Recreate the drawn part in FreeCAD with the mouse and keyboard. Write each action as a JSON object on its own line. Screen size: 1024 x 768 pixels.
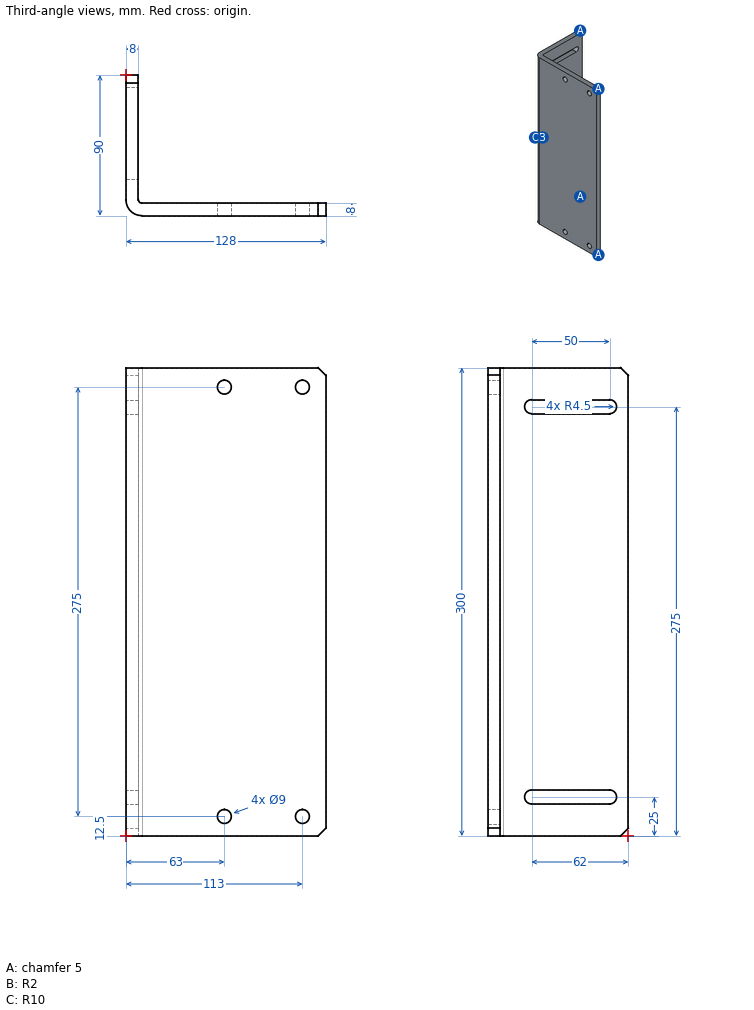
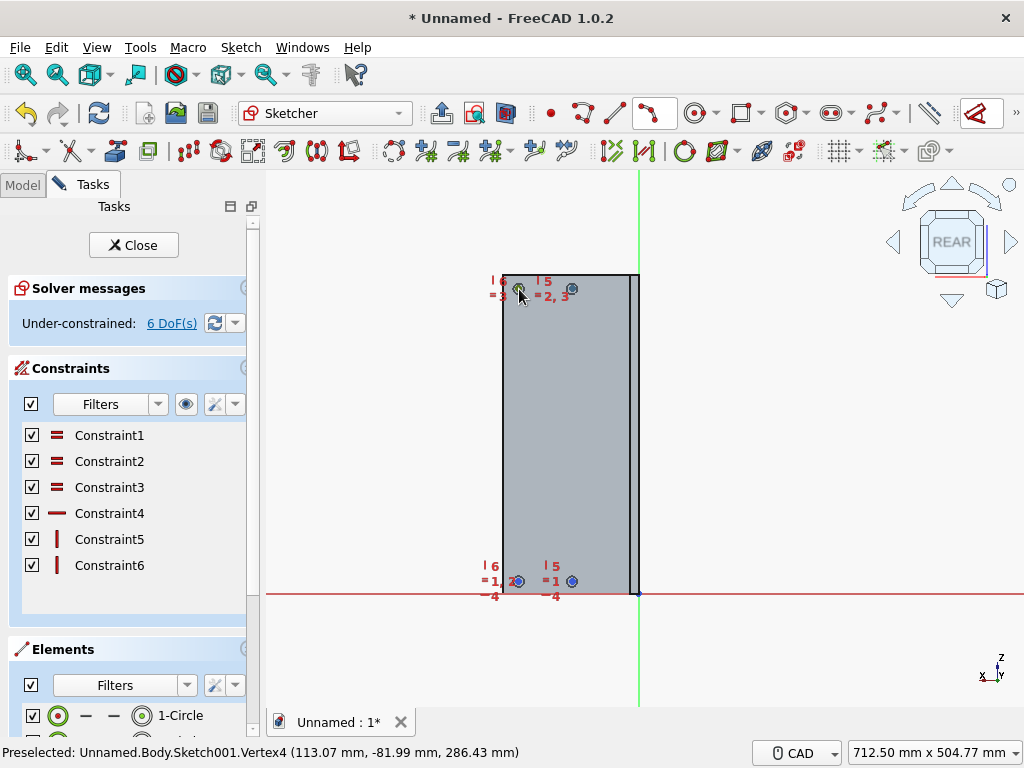
{"action": "key", "text": "h"}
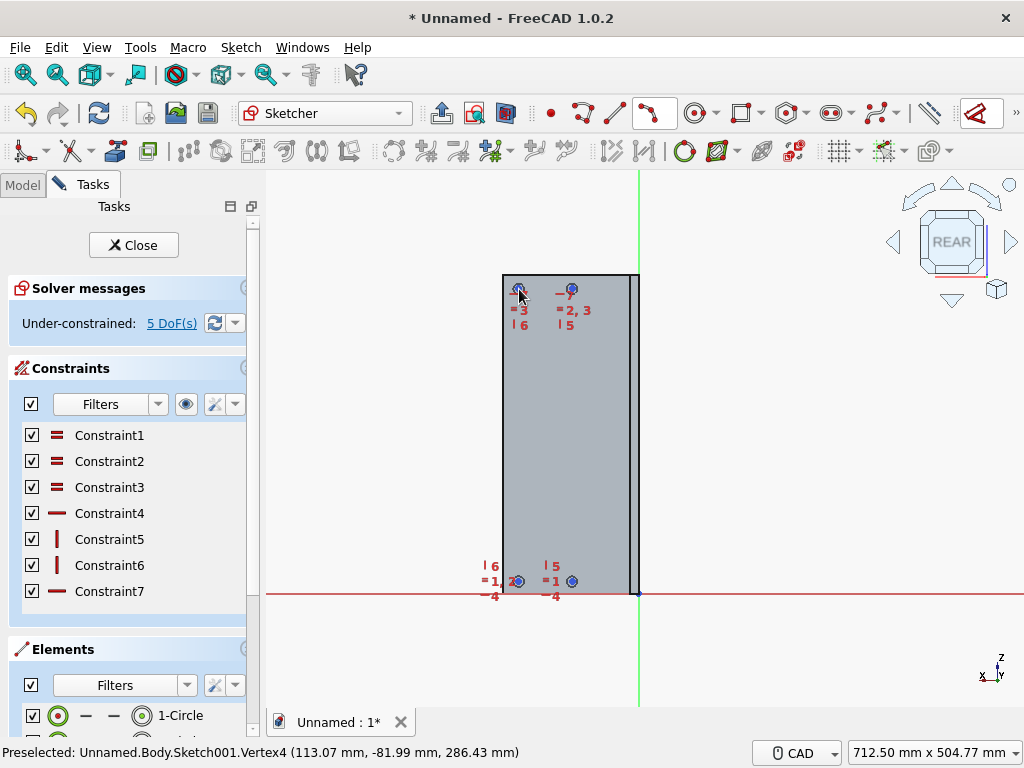
{"action": "key", "text": "d"}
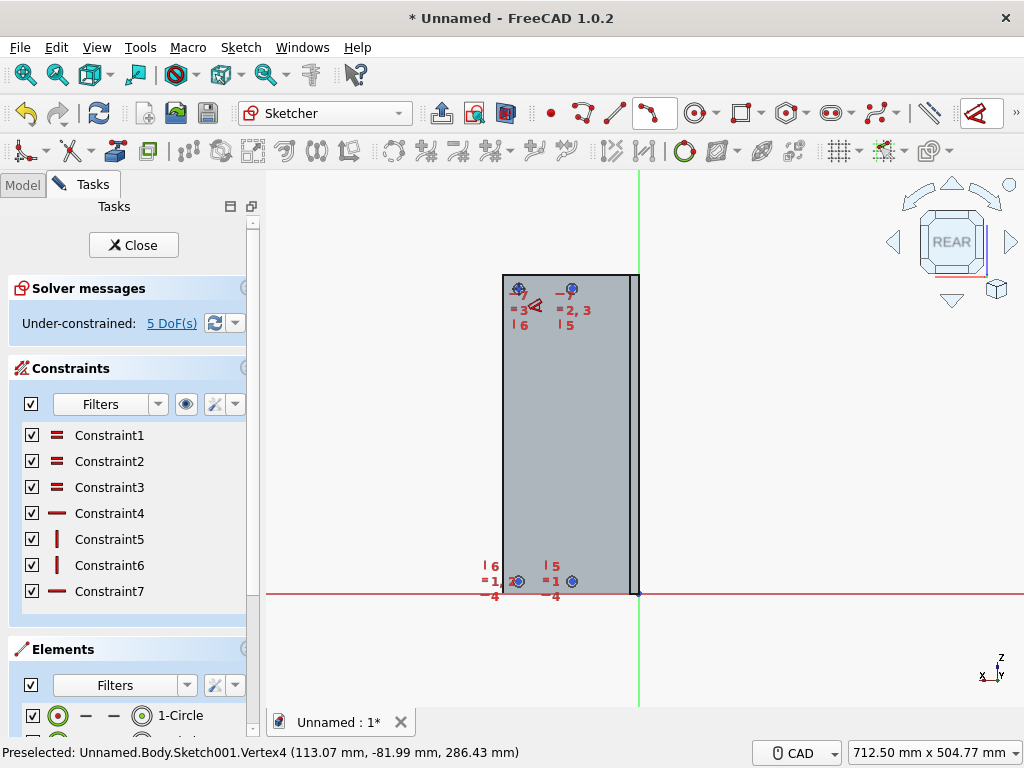
{"action": "scroll", "coordinate": [577, 582], "scroll_direction": "up", "scroll_amount": 8}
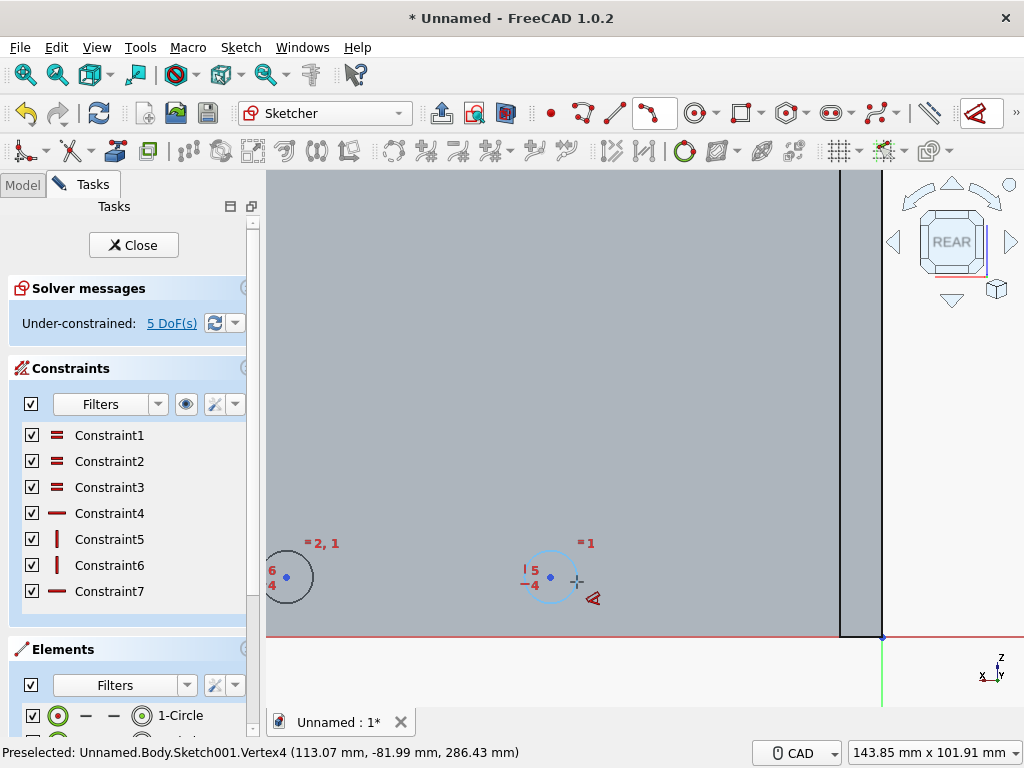
{"action": "left_click", "coordinate": [577, 578]}
{"action": "left_click", "coordinate": [609, 579]}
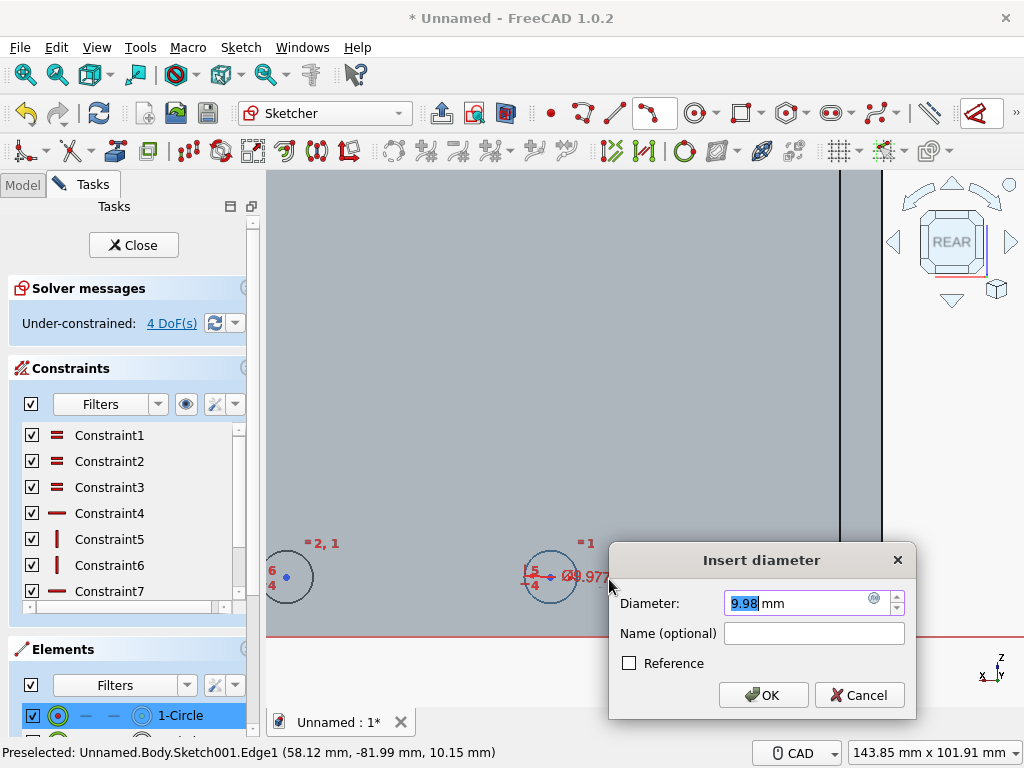
{"action": "type", "text": "9"}
{"action": "key", "text": "Return"}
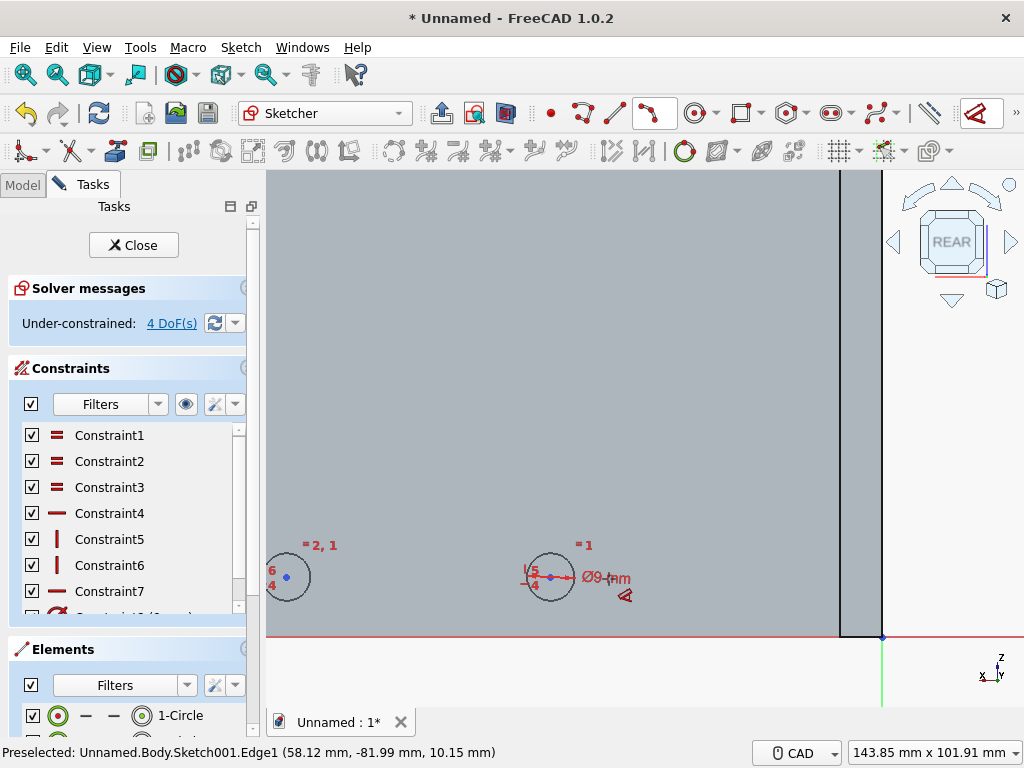
{"action": "scroll", "coordinate": [577, 583], "scroll_direction": "down", "scroll_amount": 8}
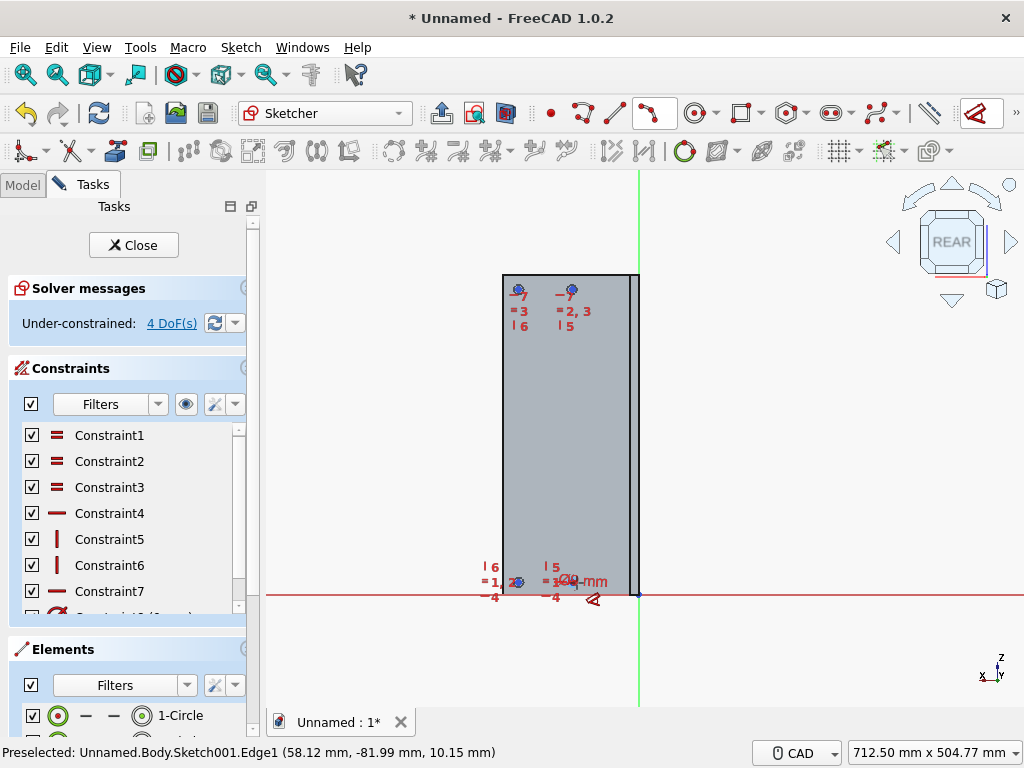
{"action": "left_click", "coordinate": [572, 582]}
{"action": "left_click", "coordinate": [606, 629]}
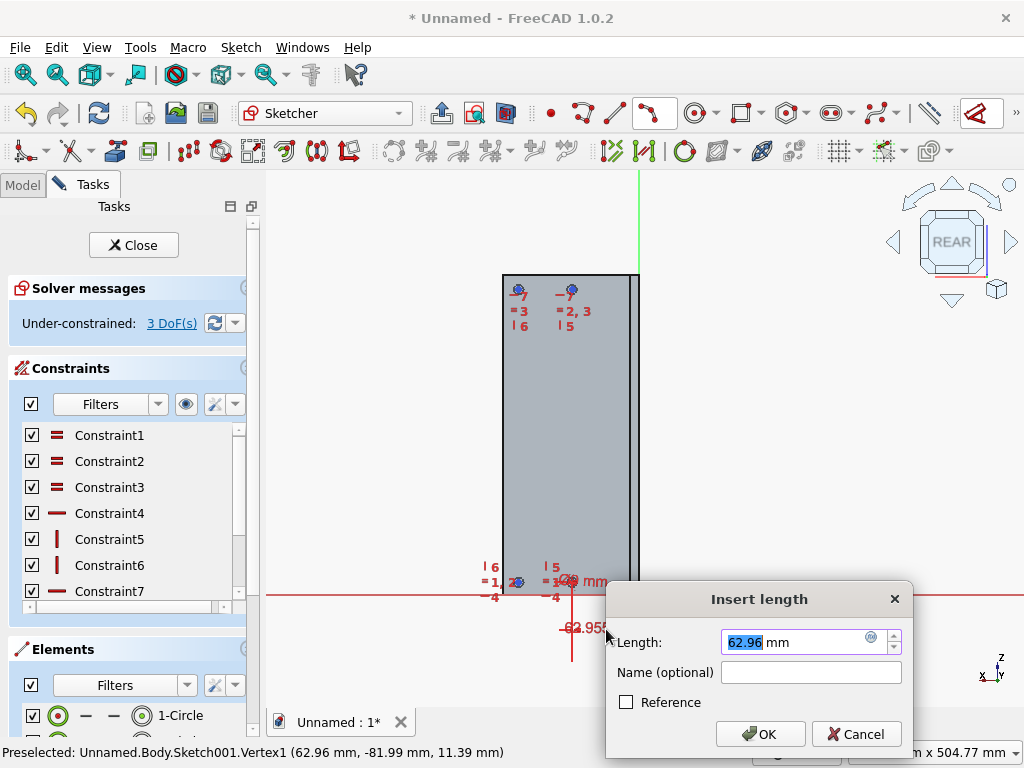
{"action": "type", "text": "63"}
{"action": "key", "text": "Return"}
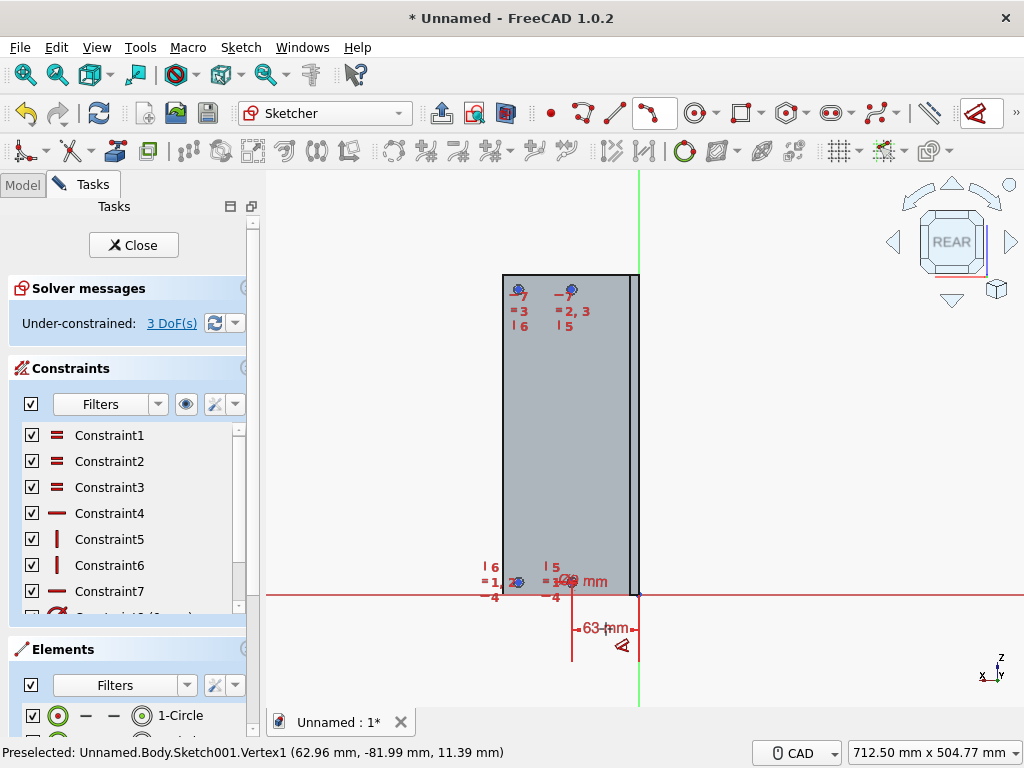
{"action": "left_click", "coordinate": [519, 582]}
{"action": "left_click", "coordinate": [579, 548]}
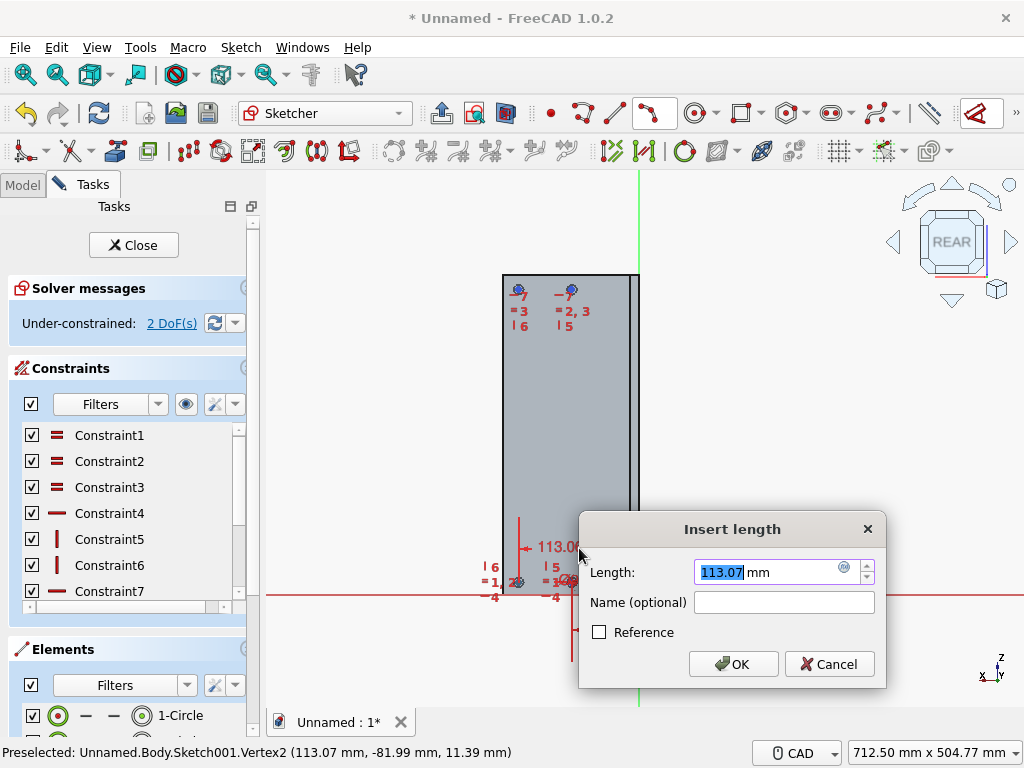
{"action": "type", "text": "113"}
{"action": "key", "text": "Return"}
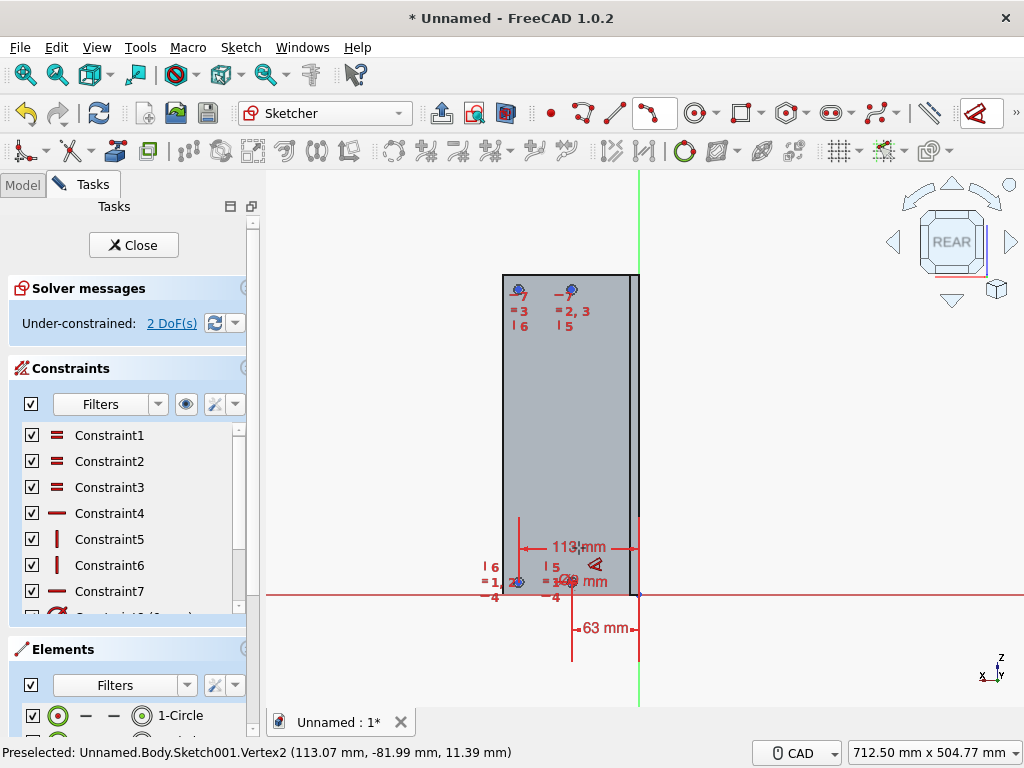
{"action": "scroll", "coordinate": [572, 582], "scroll_direction": "up", "scroll_amount": 6}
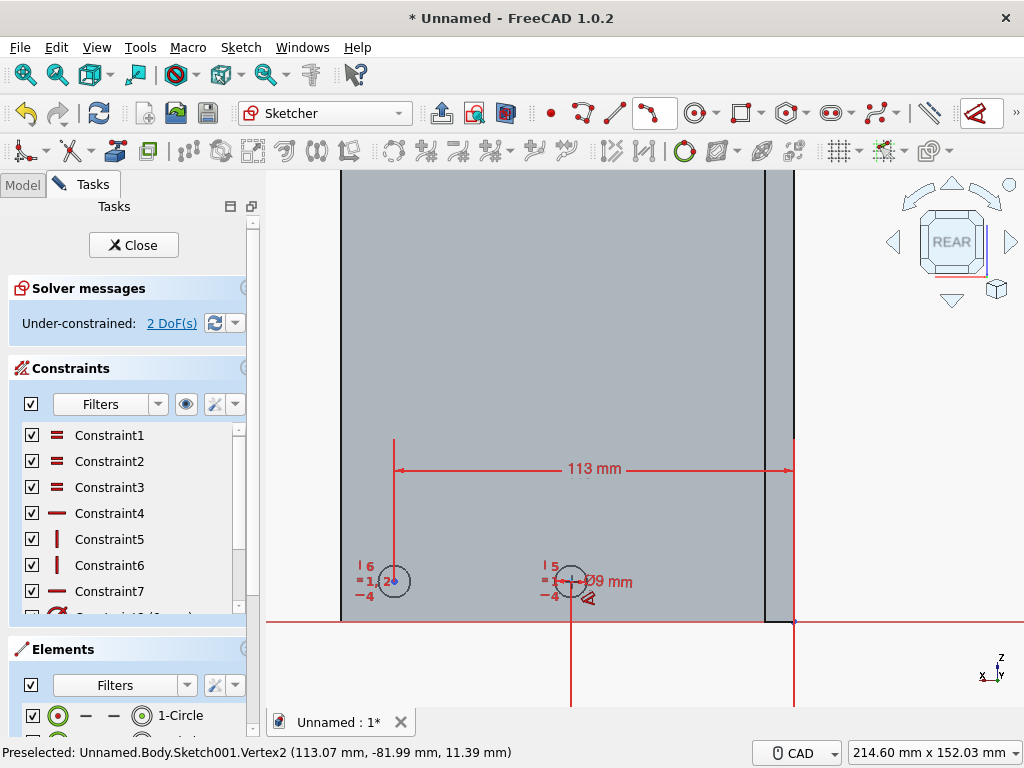
{"action": "left_click", "coordinate": [571, 582]}
{"action": "left_click", "coordinate": [828, 602]}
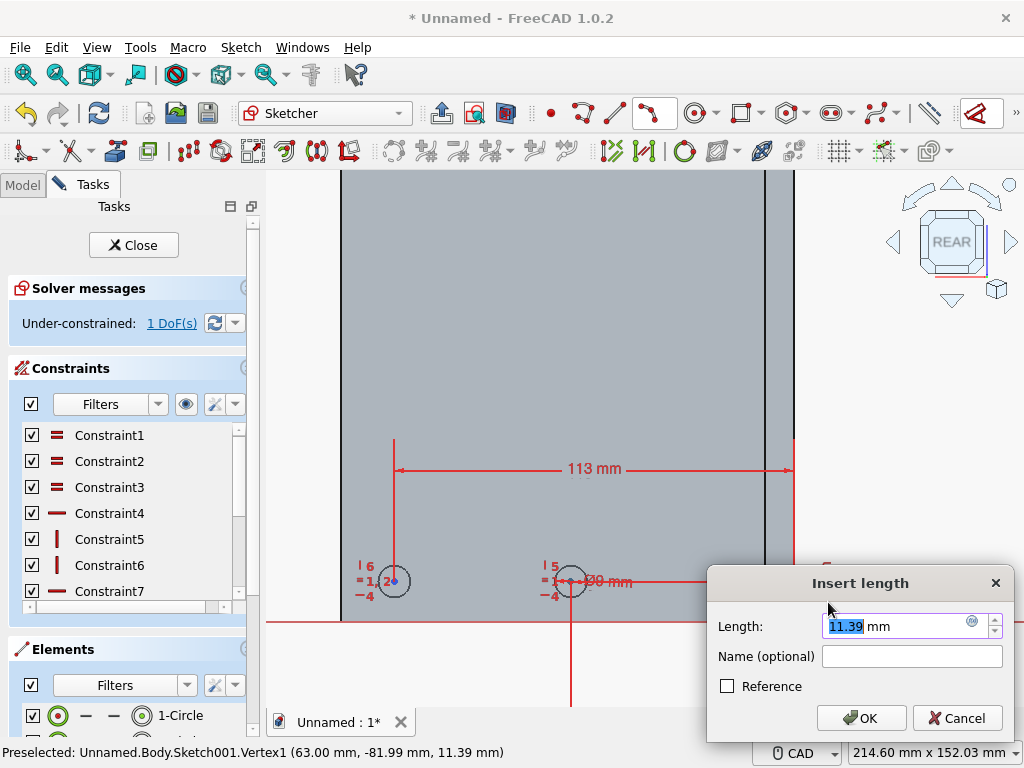
{"action": "type", "text": "12.5"}
{"action": "key", "text": "Return"}